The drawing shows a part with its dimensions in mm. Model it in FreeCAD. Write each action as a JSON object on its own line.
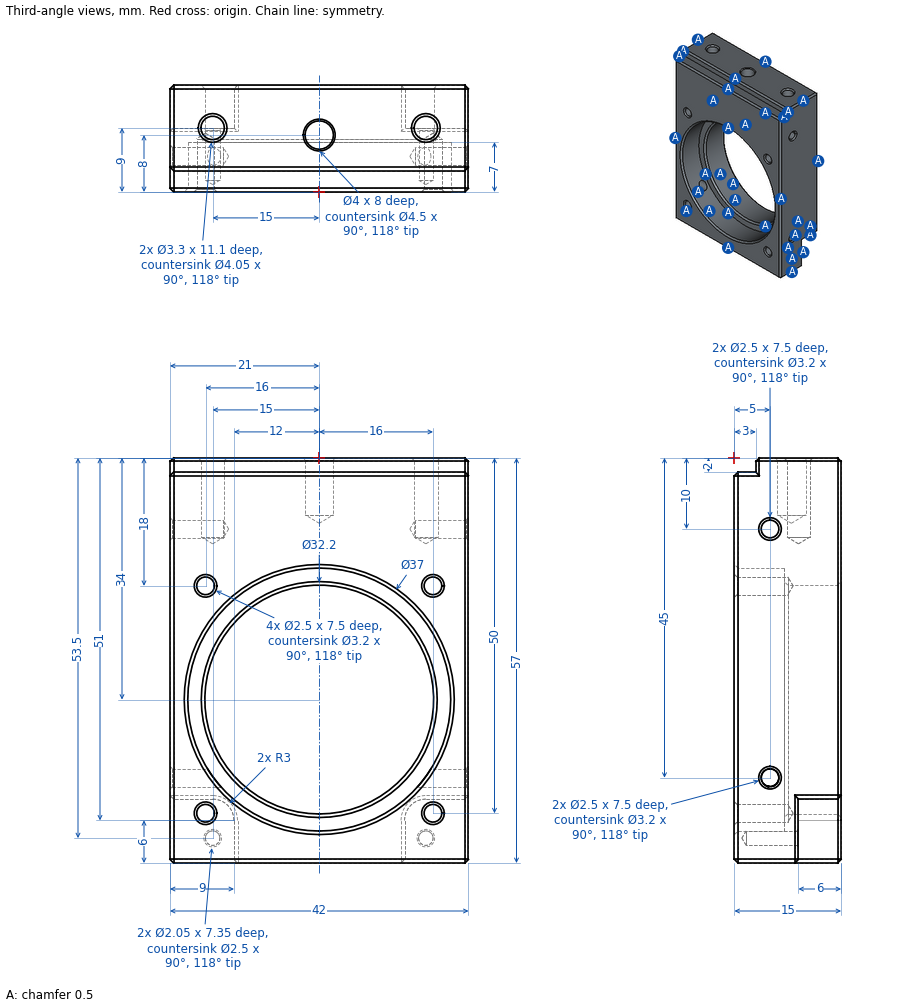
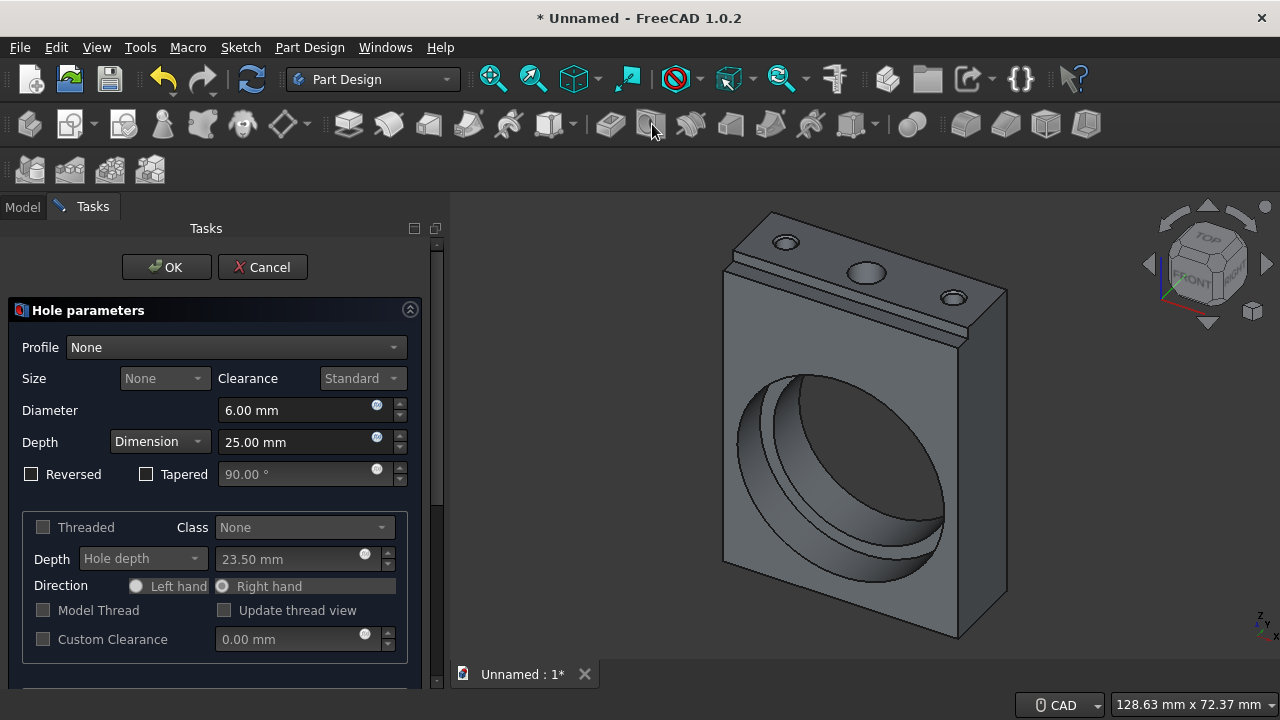
{"action": "triple_click", "coordinate": [305, 410]}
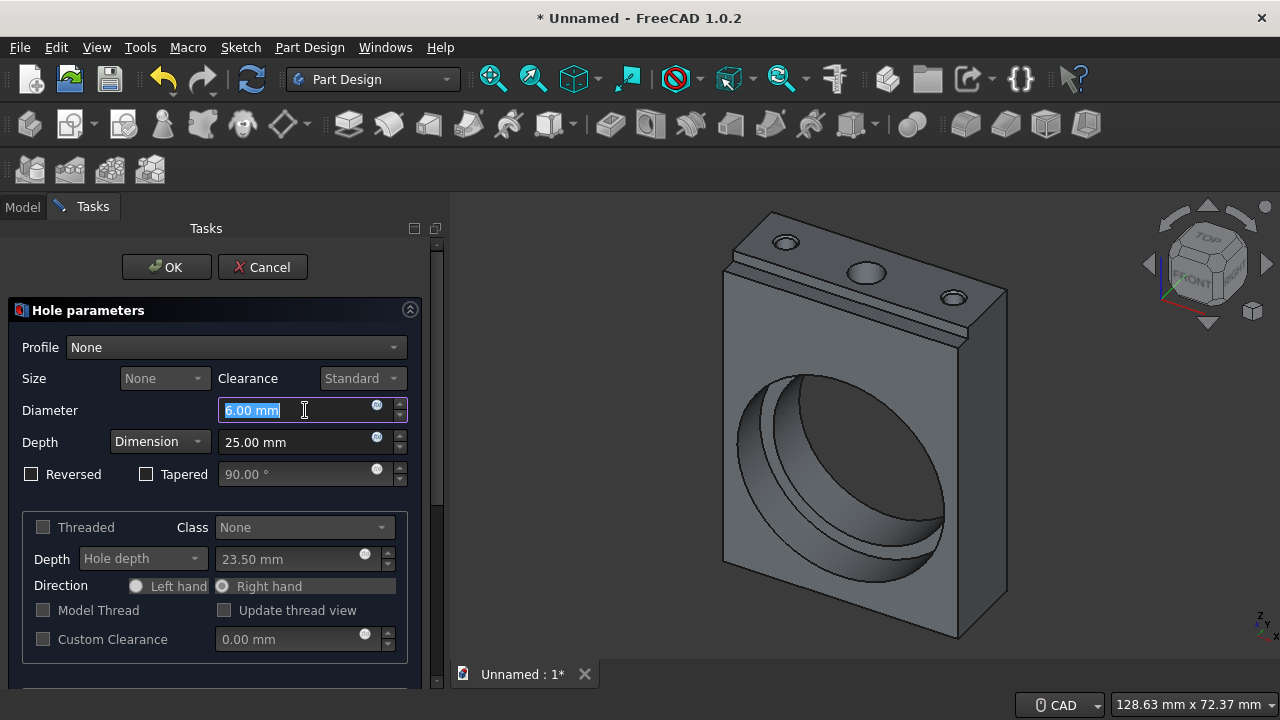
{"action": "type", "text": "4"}
{"action": "key", "text": "Tab"}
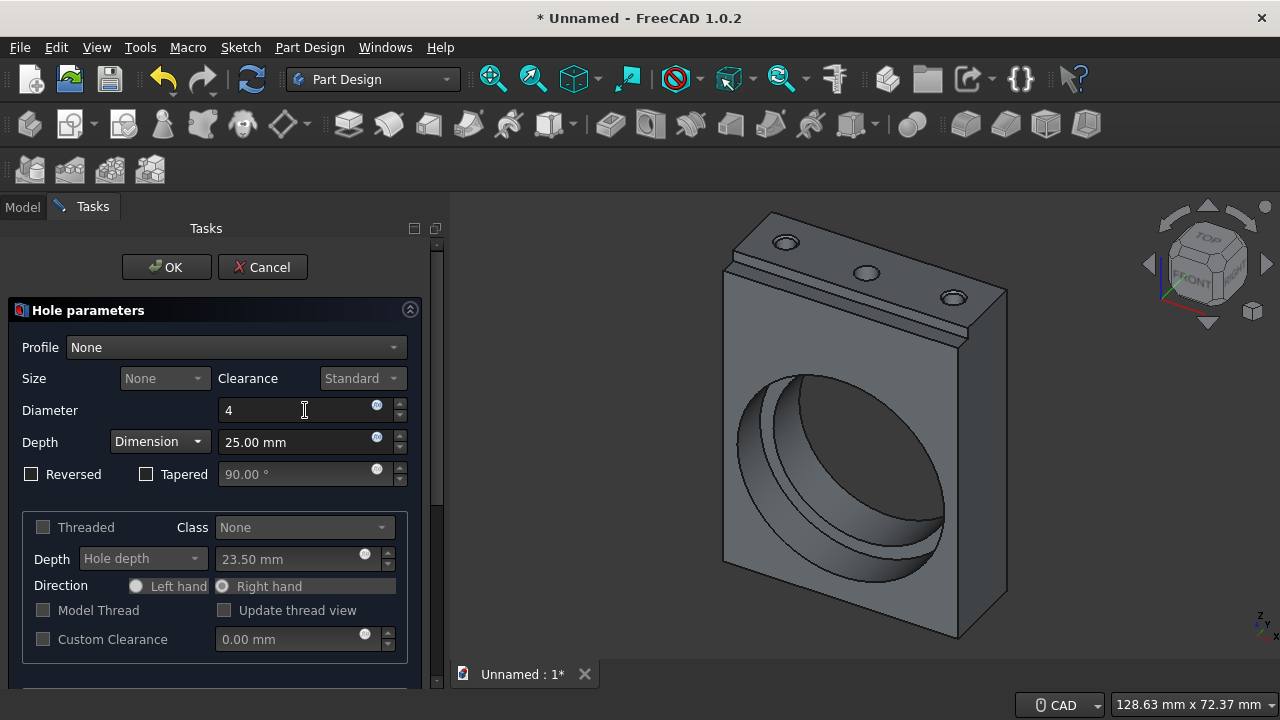
{"action": "triple_click", "coordinate": [305, 442]}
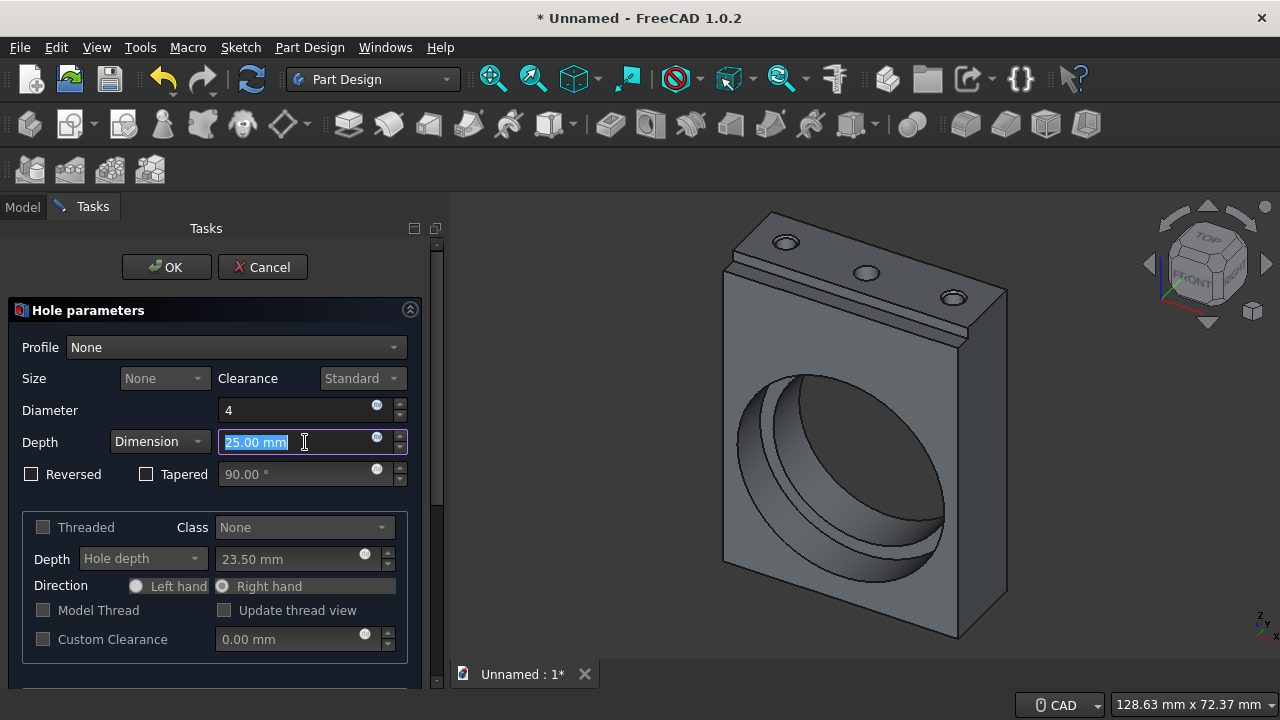
{"action": "type", "text": "8"}
{"action": "key", "text": "Tab"}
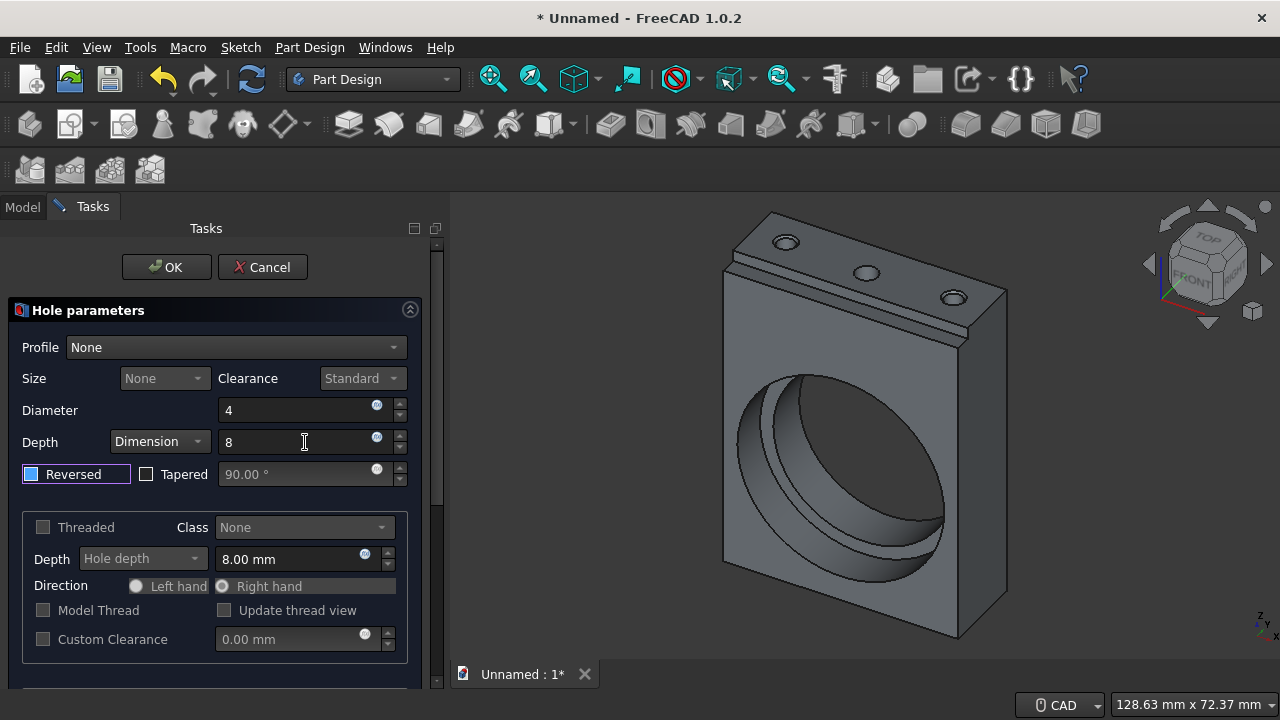
{"action": "scroll", "coordinate": [437, 463], "scroll_direction": "down", "scroll_amount": 2}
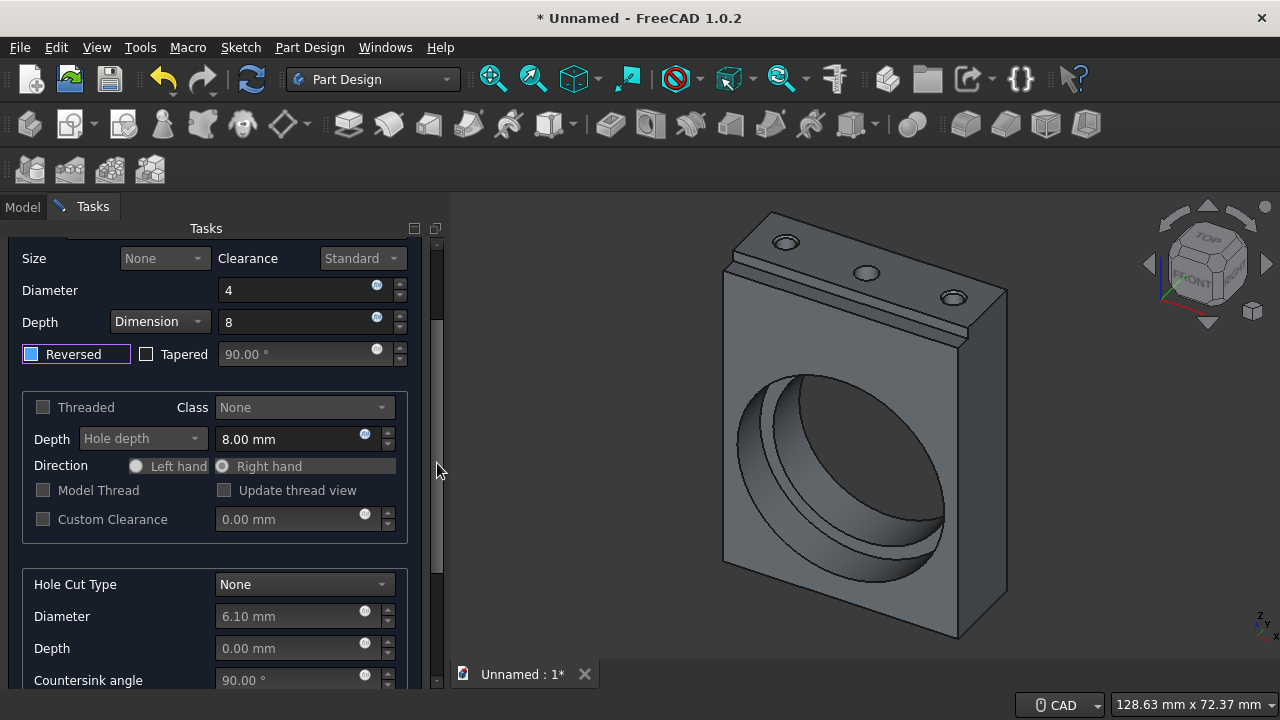
{"action": "left_click", "coordinate": [306, 584]}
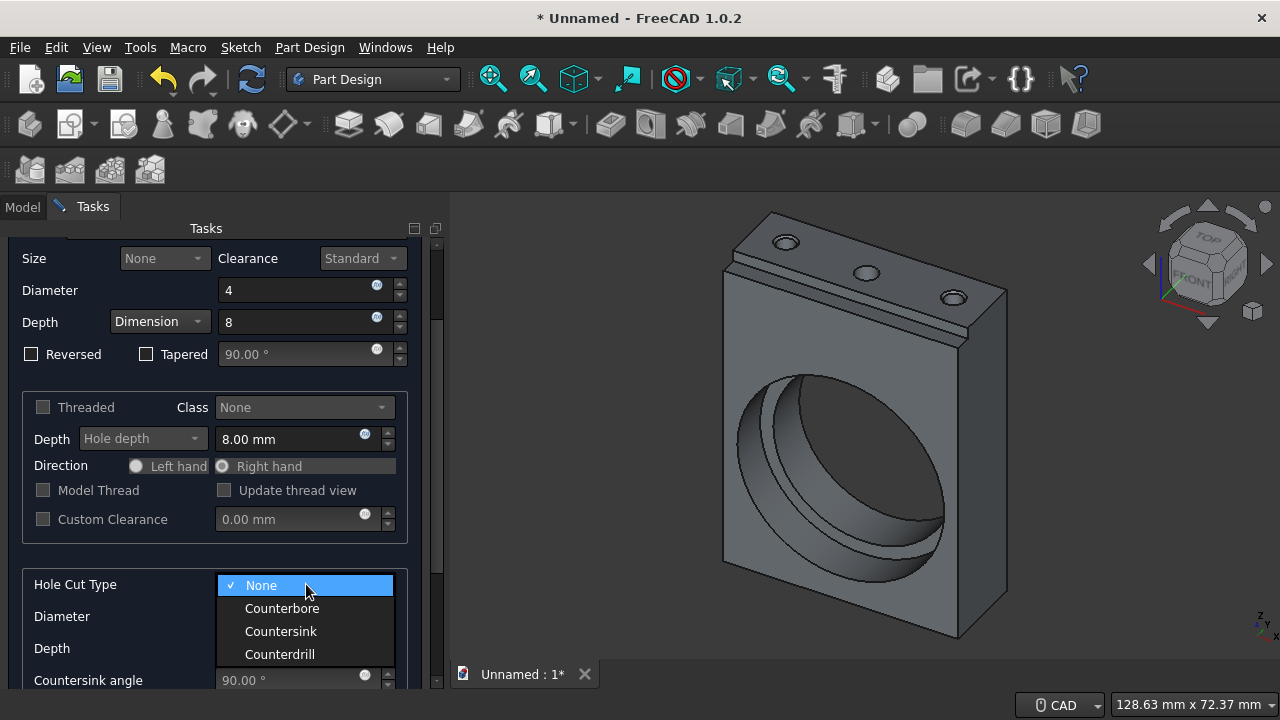
{"action": "left_click", "coordinate": [304, 632]}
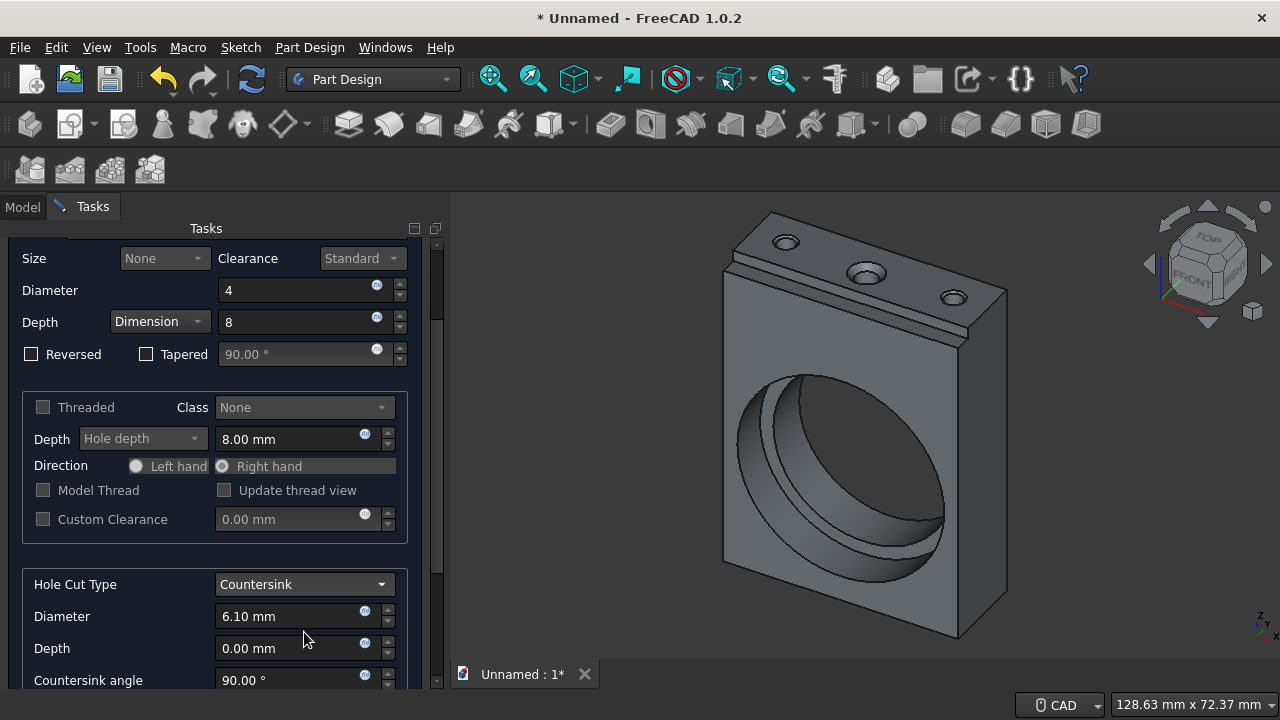
{"action": "triple_click", "coordinate": [298, 616]}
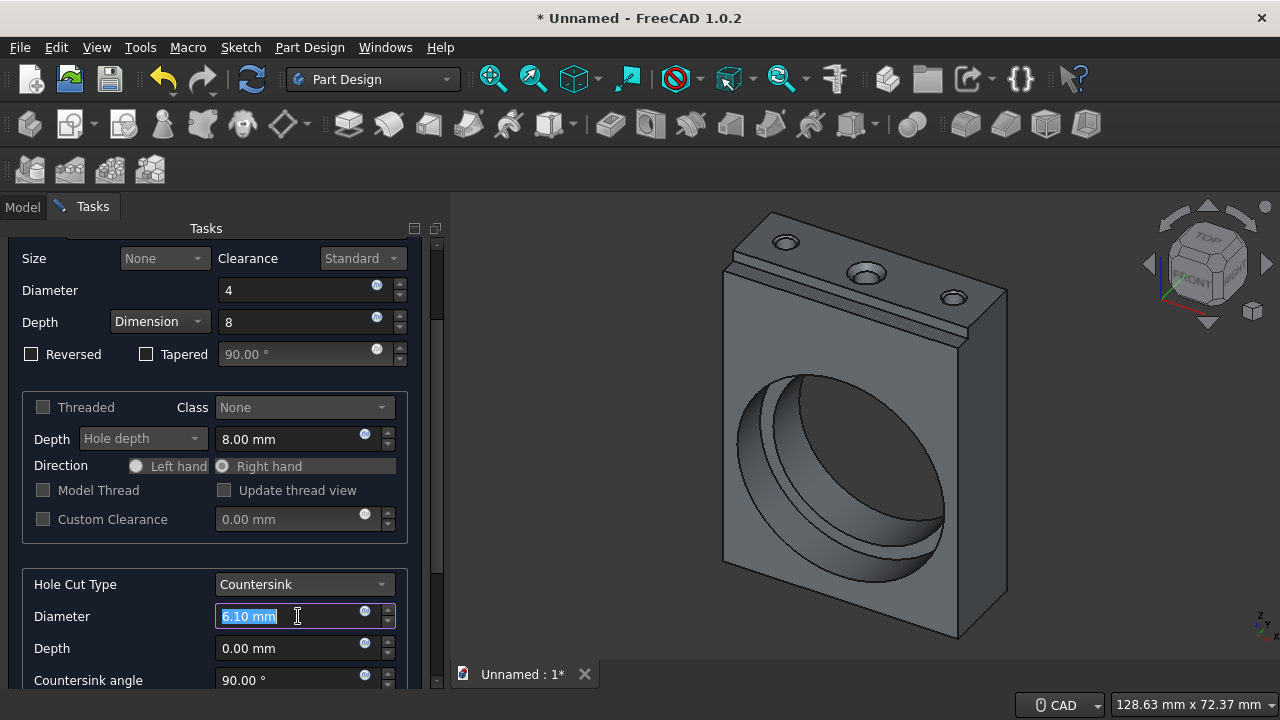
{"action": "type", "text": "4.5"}
{"action": "key", "text": "Tab"}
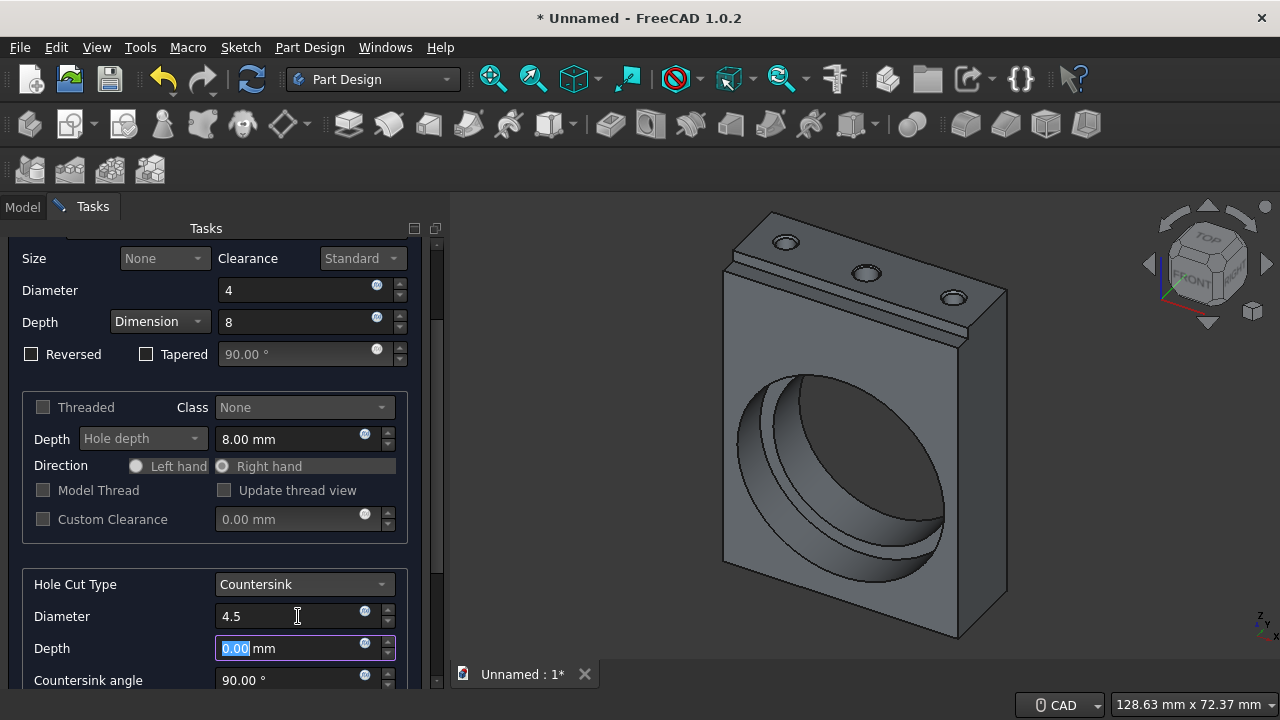
{"action": "scroll", "coordinate": [437, 463], "scroll_direction": "up", "scroll_amount": 3}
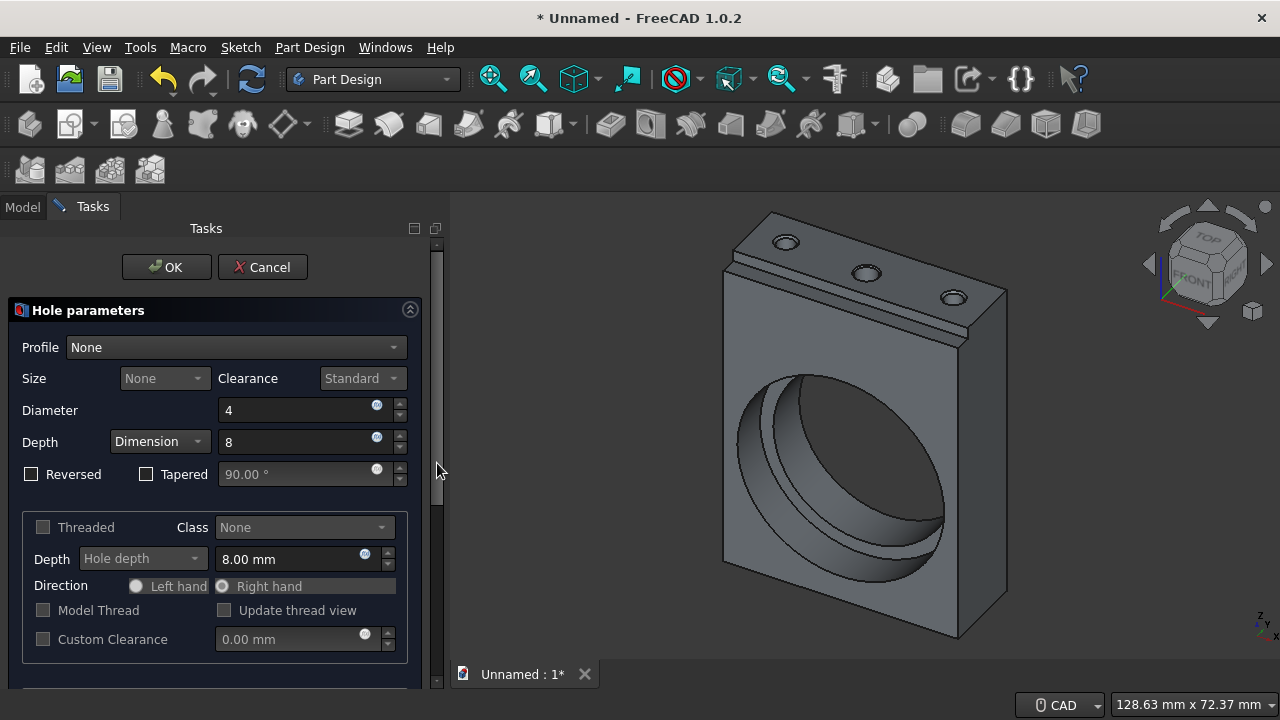
{"action": "left_click", "coordinate": [167, 267]}